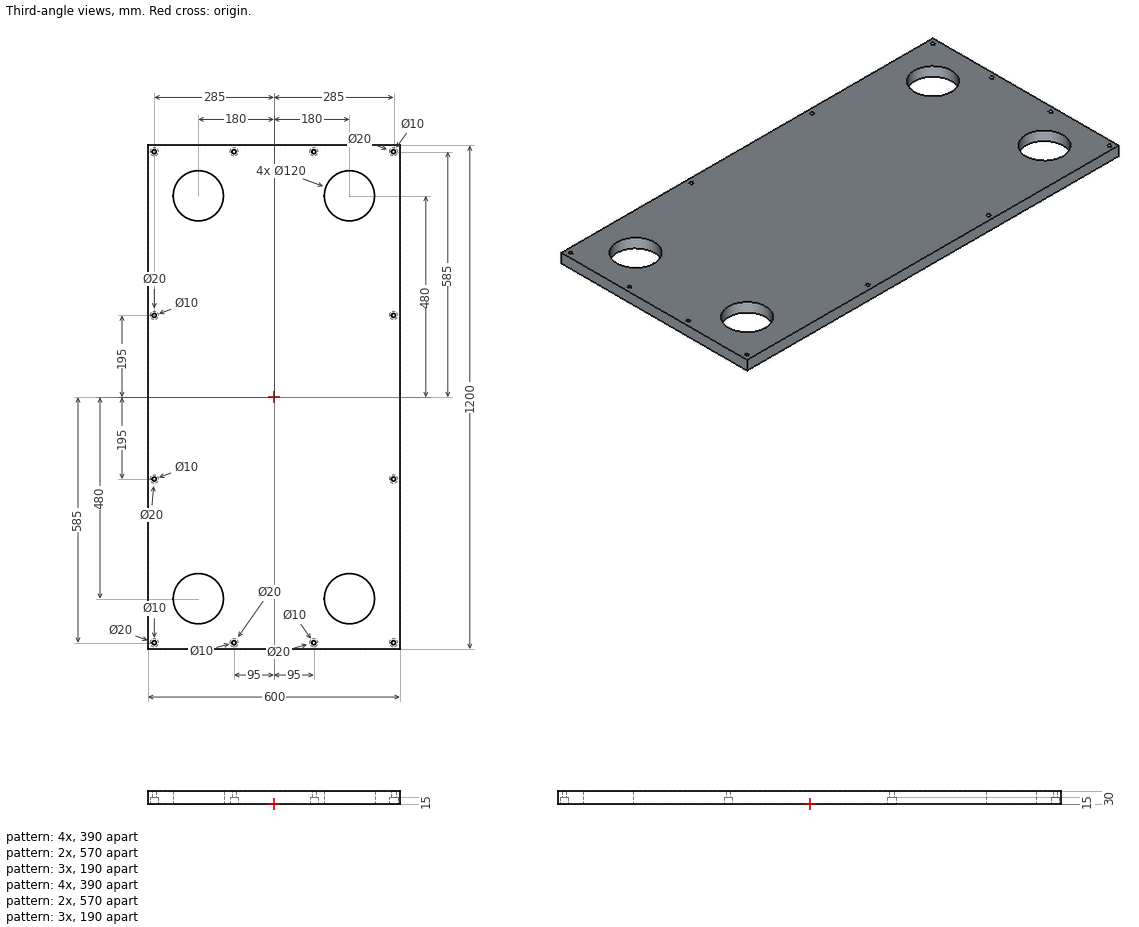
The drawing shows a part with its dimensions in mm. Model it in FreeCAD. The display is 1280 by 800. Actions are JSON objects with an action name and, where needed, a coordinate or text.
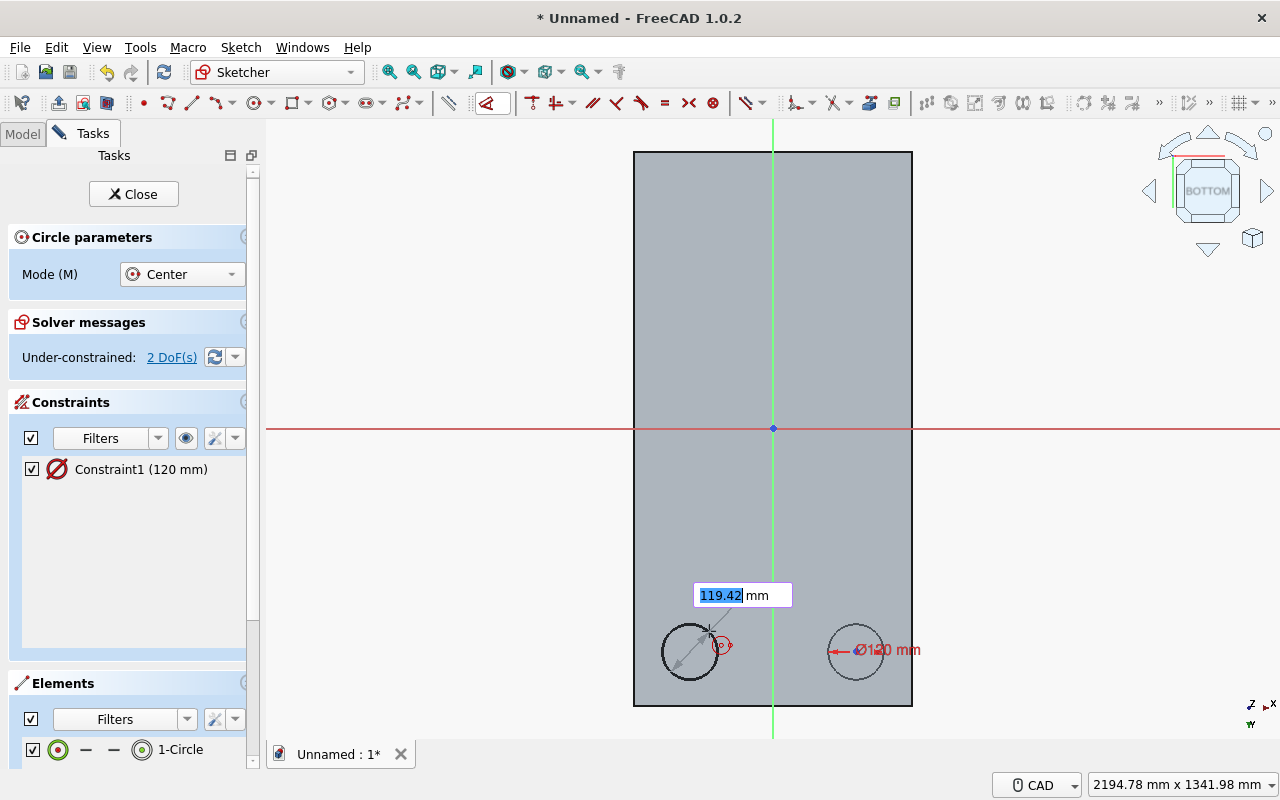
{"action": "type", "text": "120"}
{"action": "key", "text": "Return"}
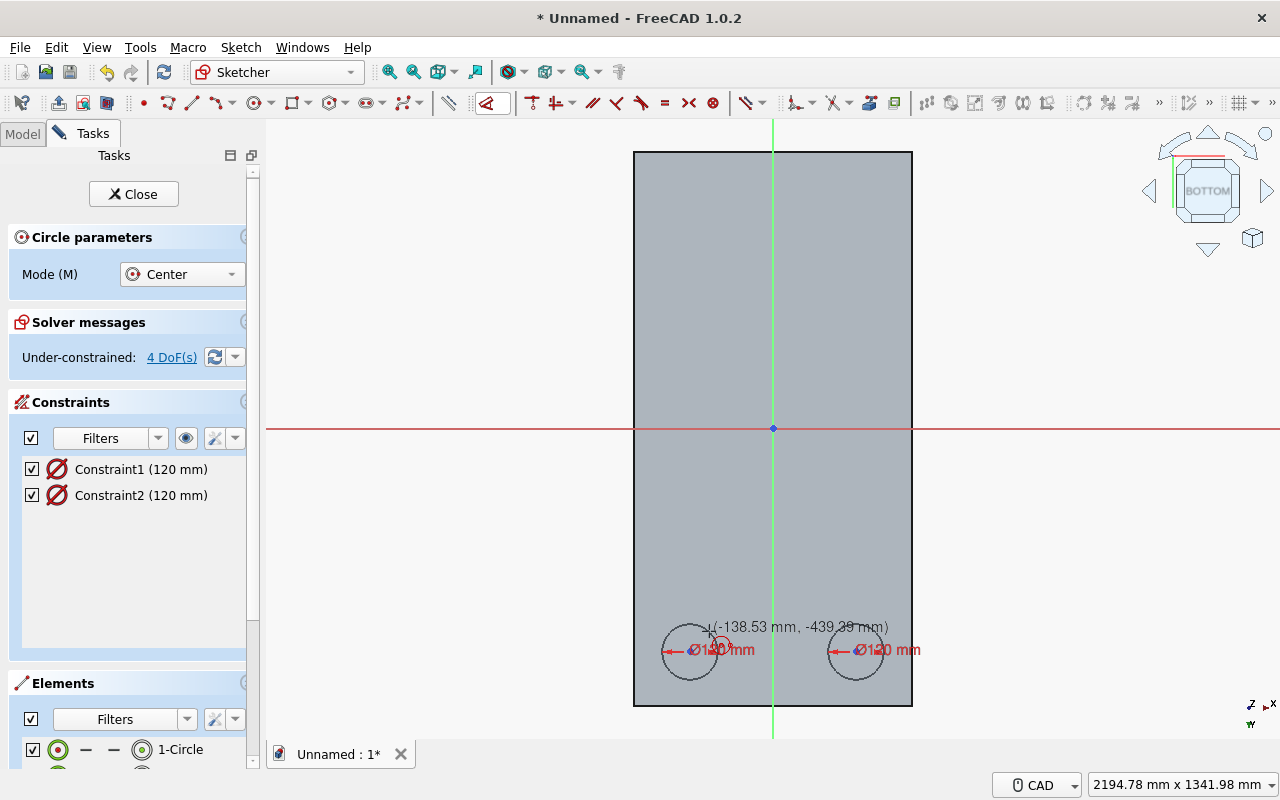
{"action": "left_click", "coordinate": [690, 207]}
{"action": "mouse_move", "coordinate": [709, 188]}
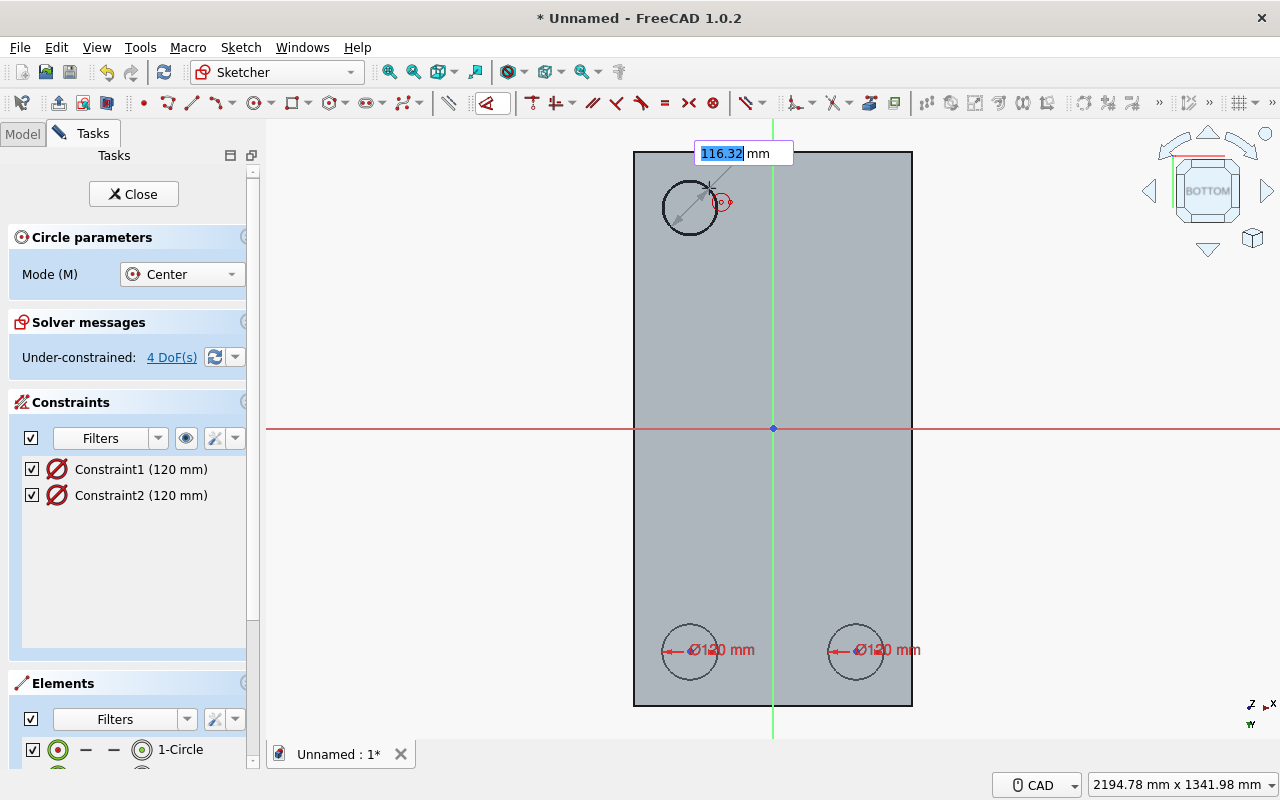
{"action": "type", "text": "120"}
{"action": "key", "text": "Return"}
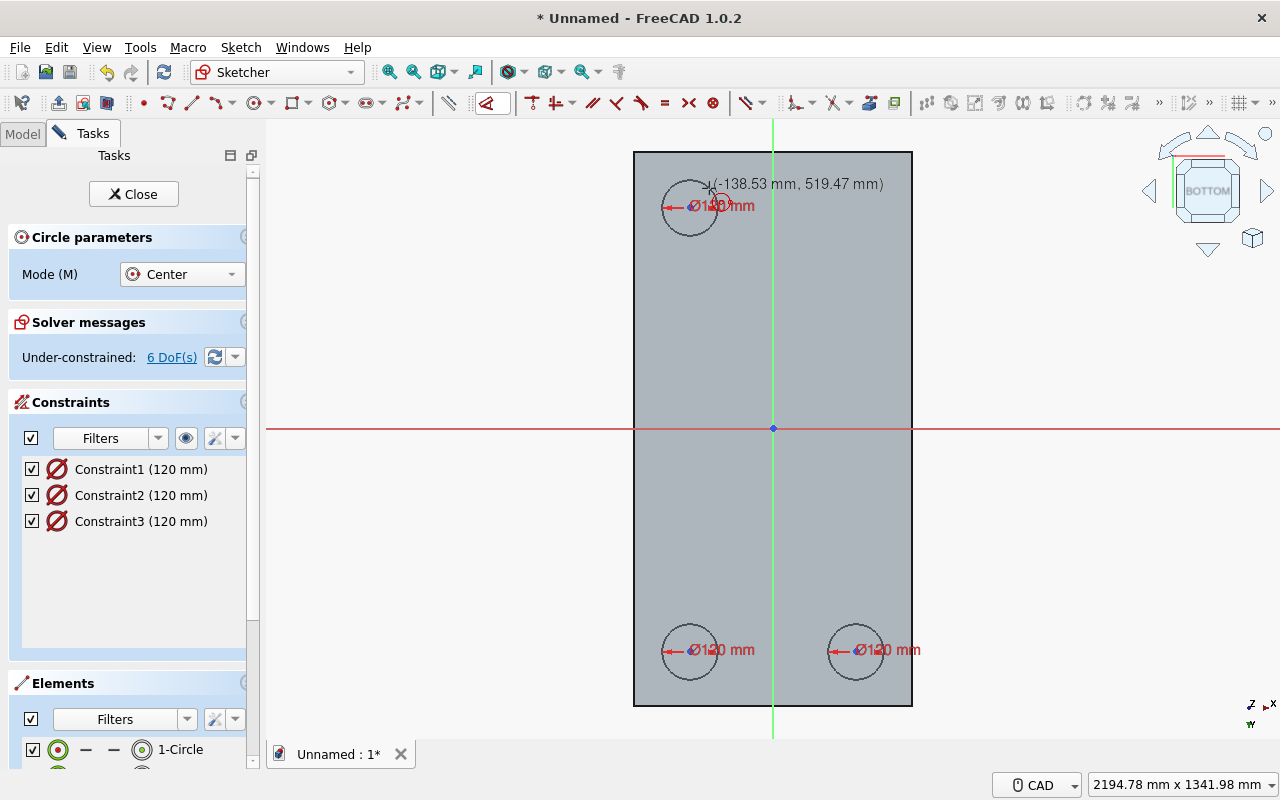
{"action": "left_click", "coordinate": [856, 207]}
{"action": "mouse_move", "coordinate": [876, 188]}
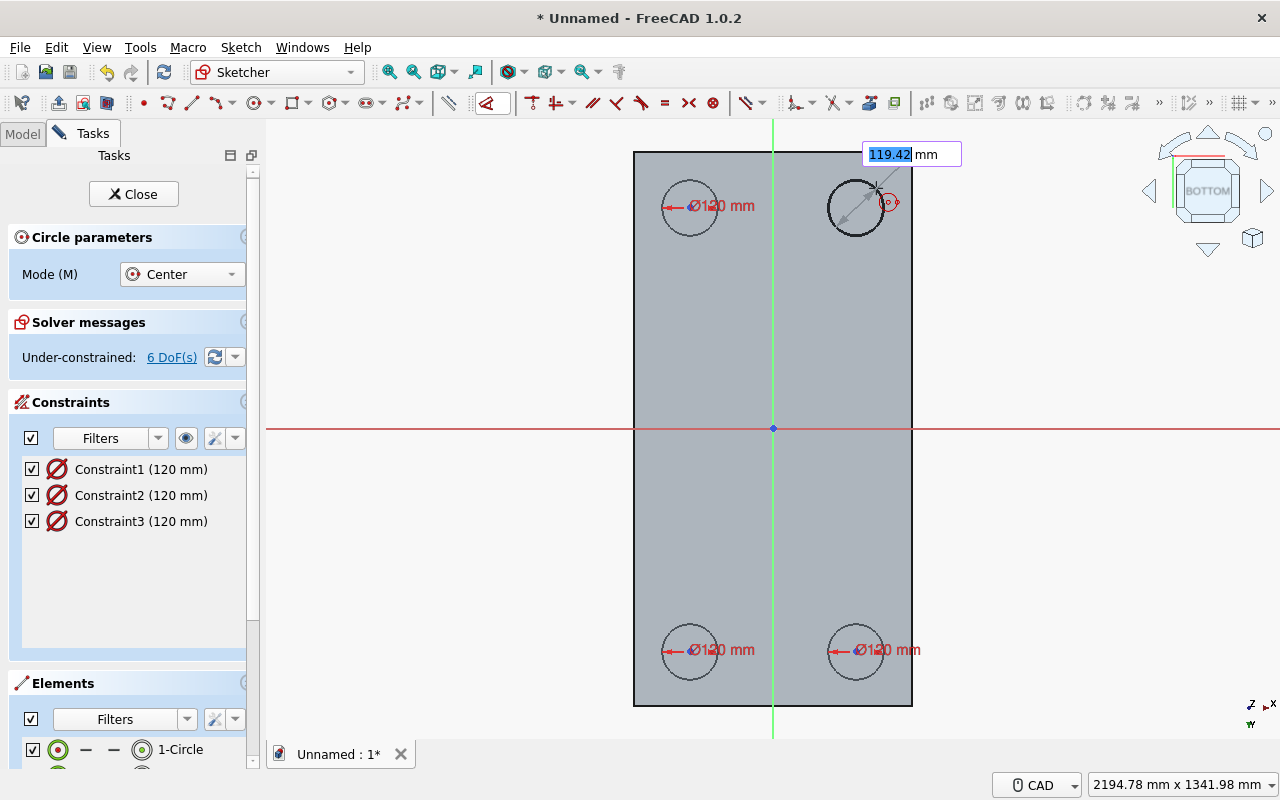
{"action": "type", "text": "120"}
{"action": "key", "text": "Return"}
{"action": "key", "text": "Escape"}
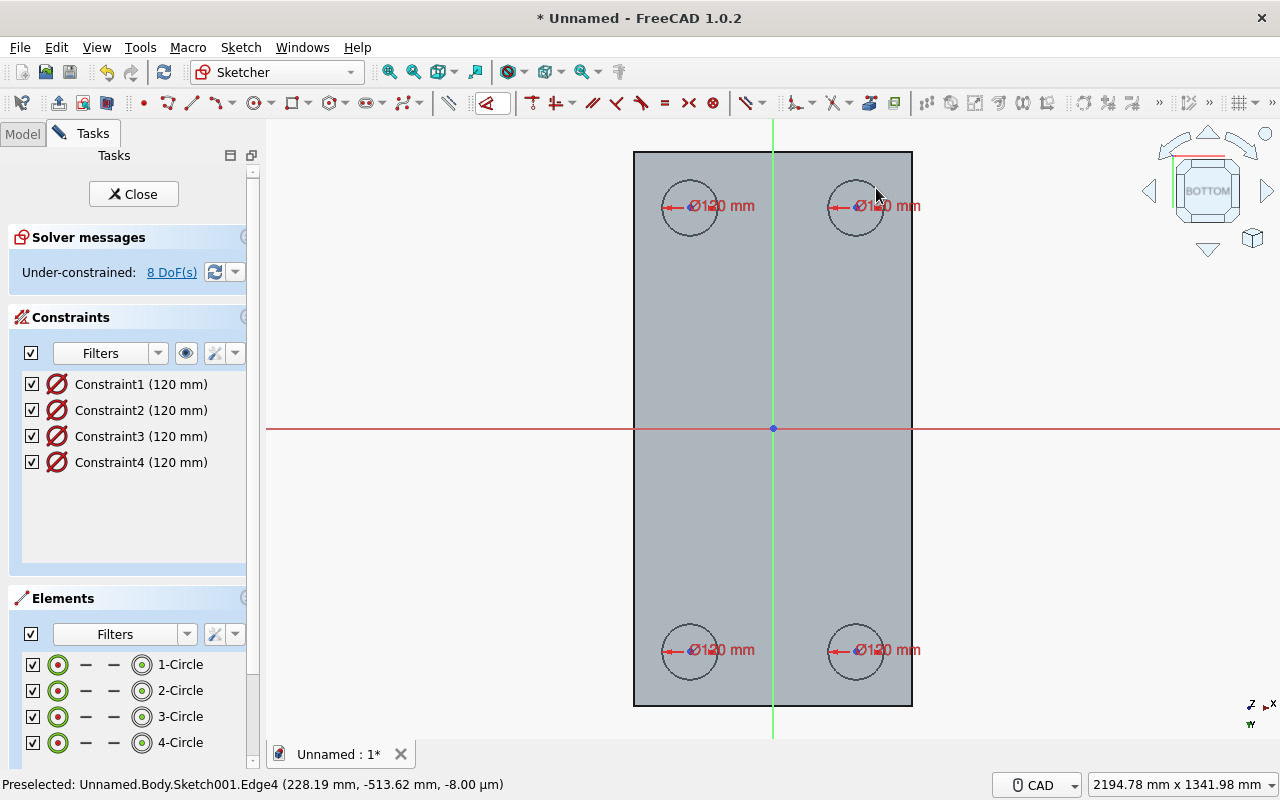
{"action": "left_click", "coordinate": [486, 104]}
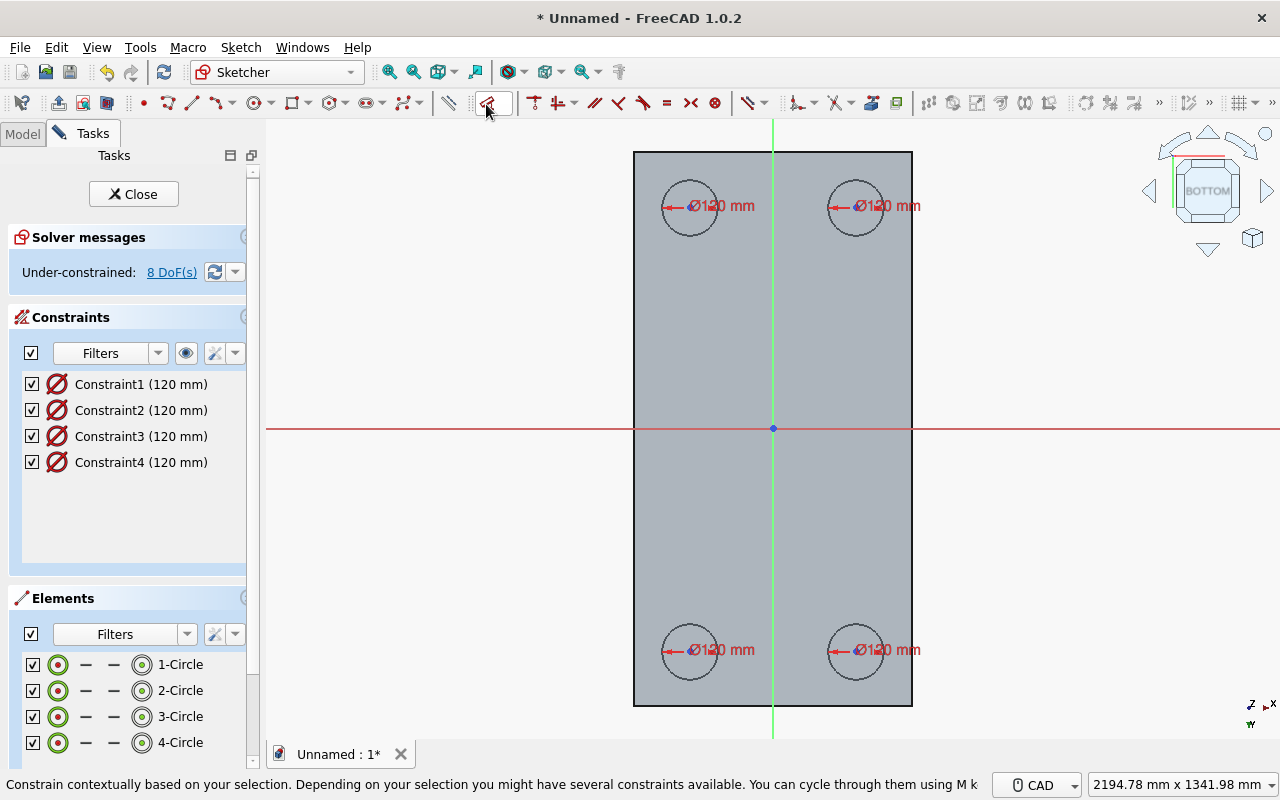
{"action": "left_click", "coordinate": [856, 652]}
{"action": "left_click", "coordinate": [814, 686]}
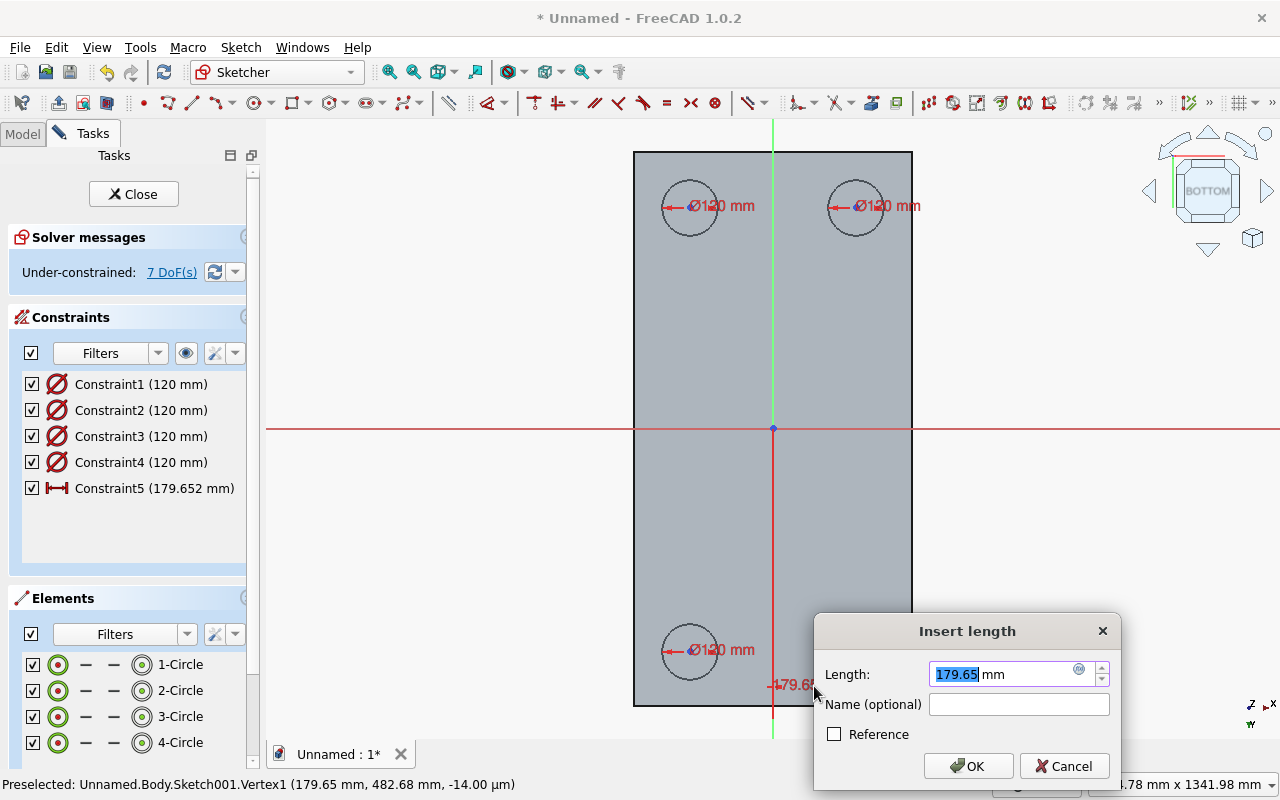
{"action": "type", "text": "180"}
{"action": "key", "text": "Return"}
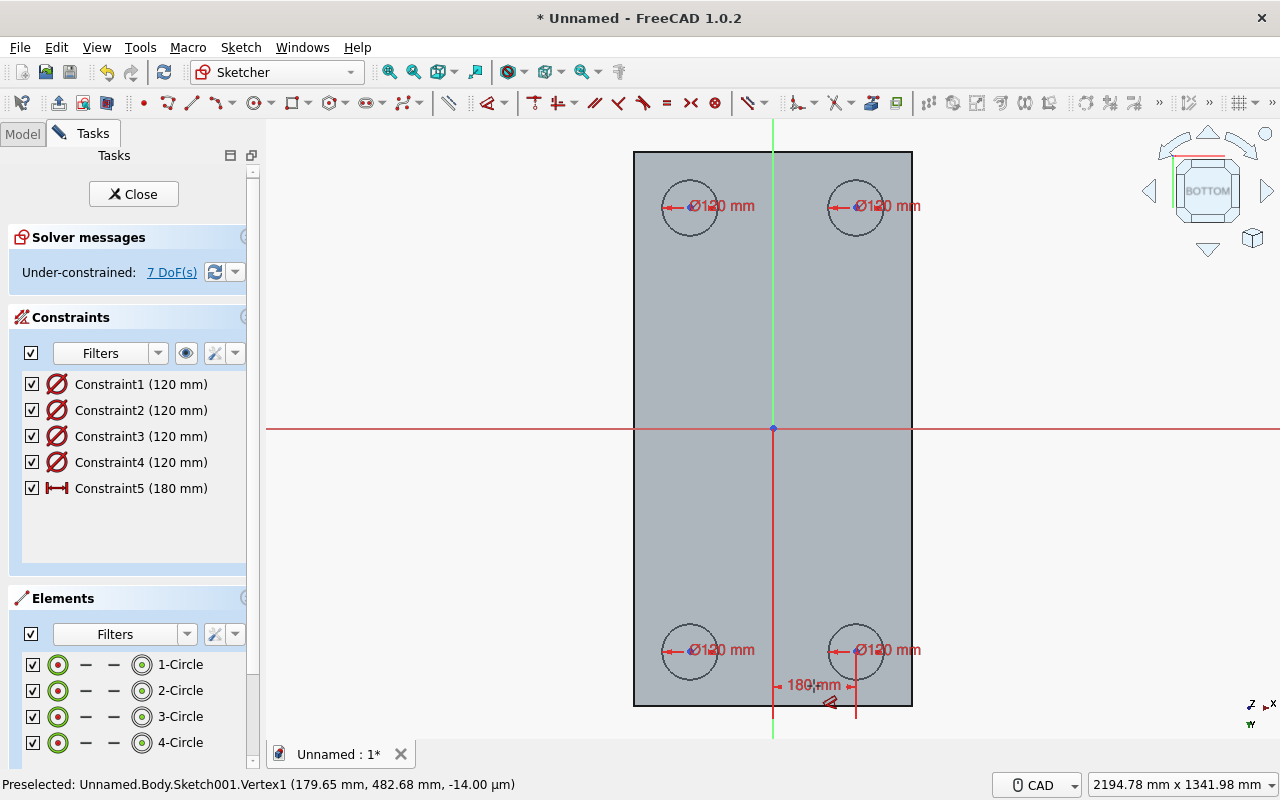
{"action": "left_click", "coordinate": [856, 652]}
{"action": "left_click", "coordinate": [890, 540]}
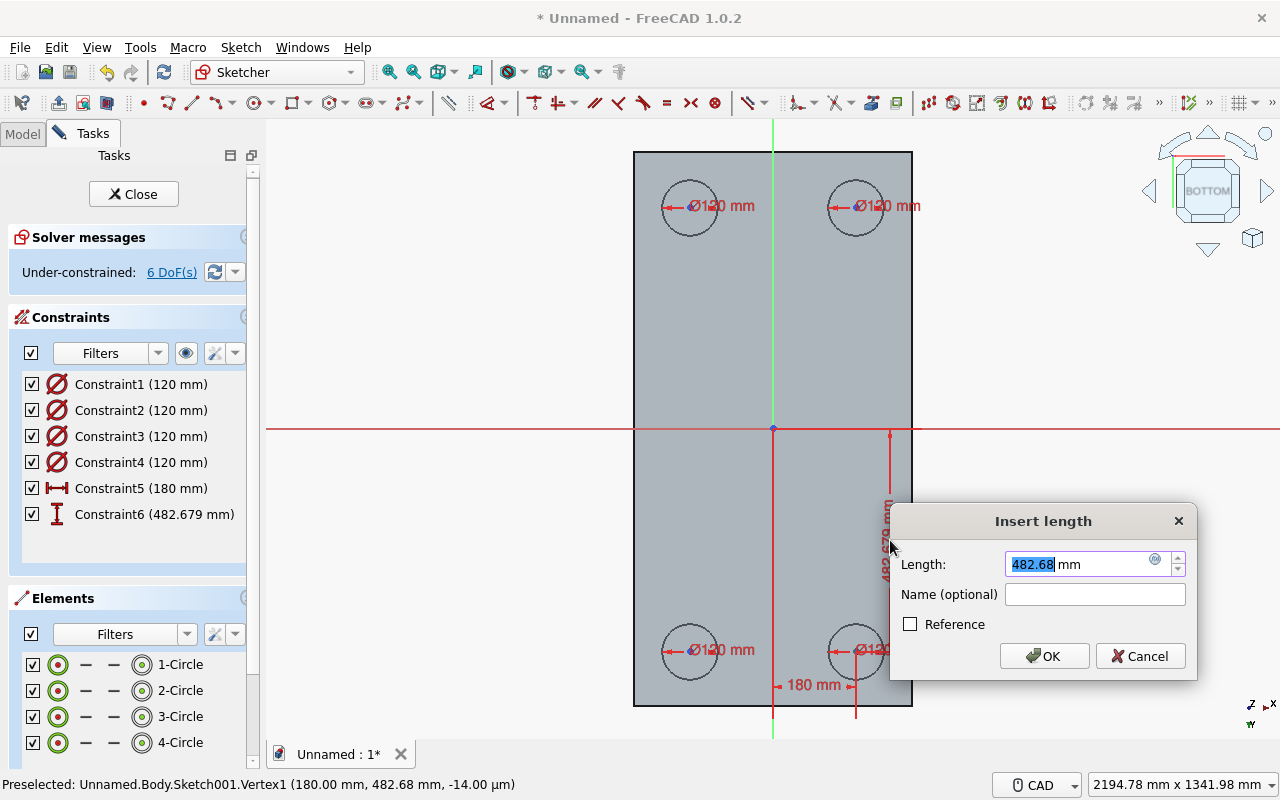
{"action": "type", "text": "480"}
{"action": "key", "text": "Return"}